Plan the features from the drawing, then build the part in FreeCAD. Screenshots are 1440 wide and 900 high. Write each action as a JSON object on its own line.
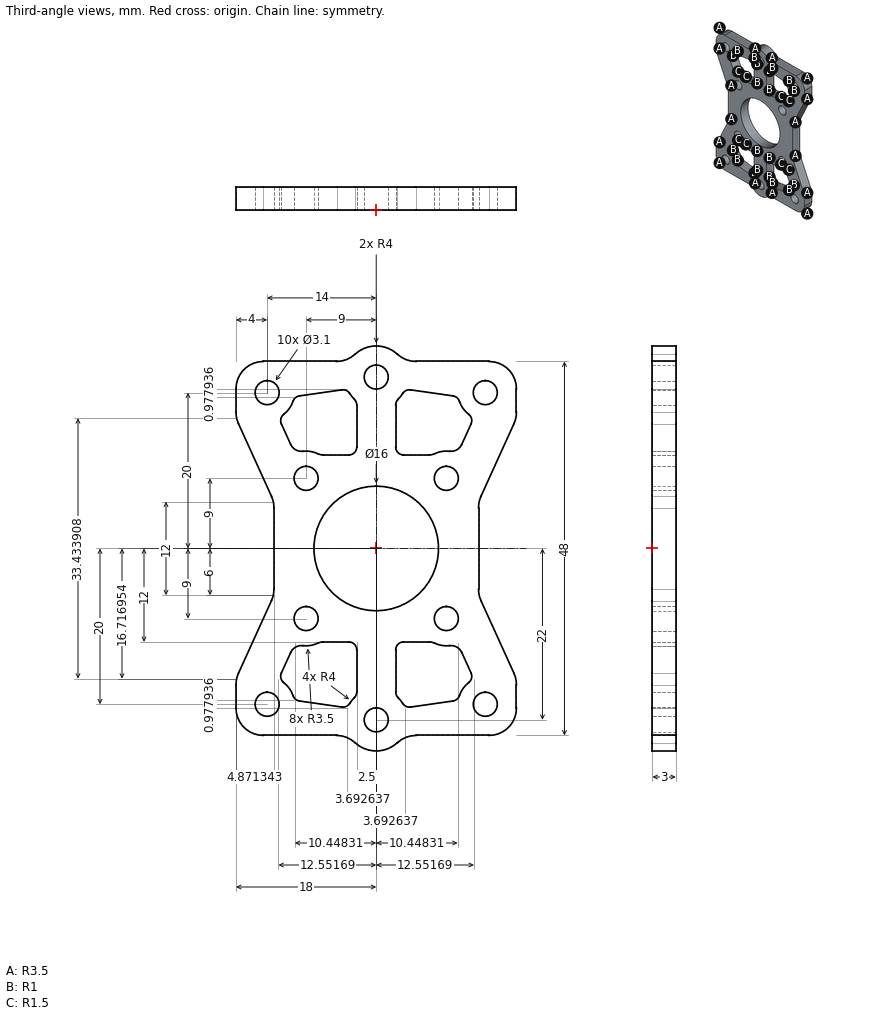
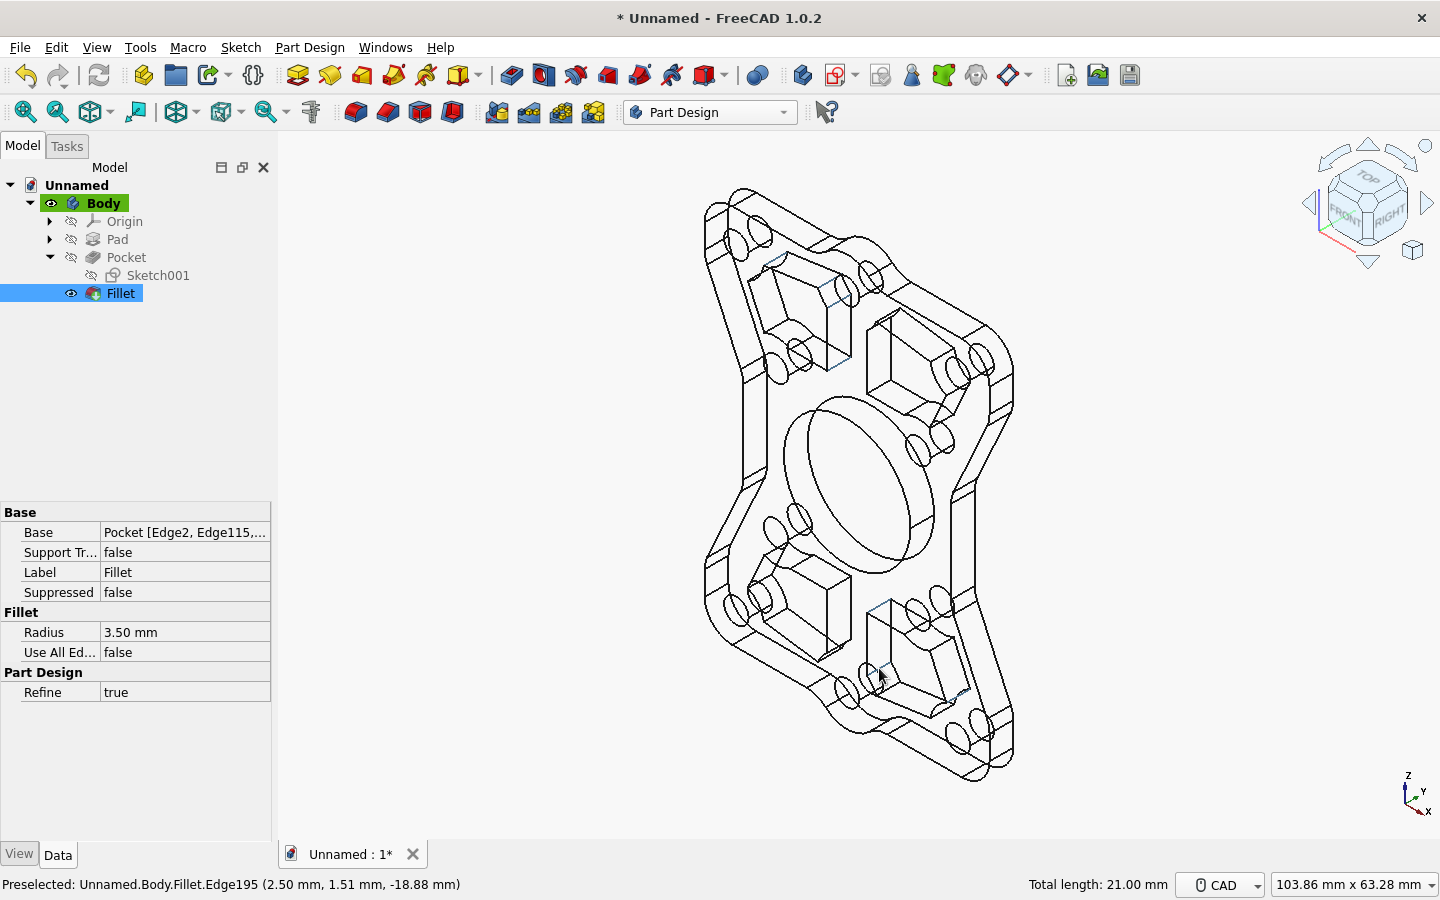
{"action": "left_click", "coordinate": [888, 688], "text": "ctrl"}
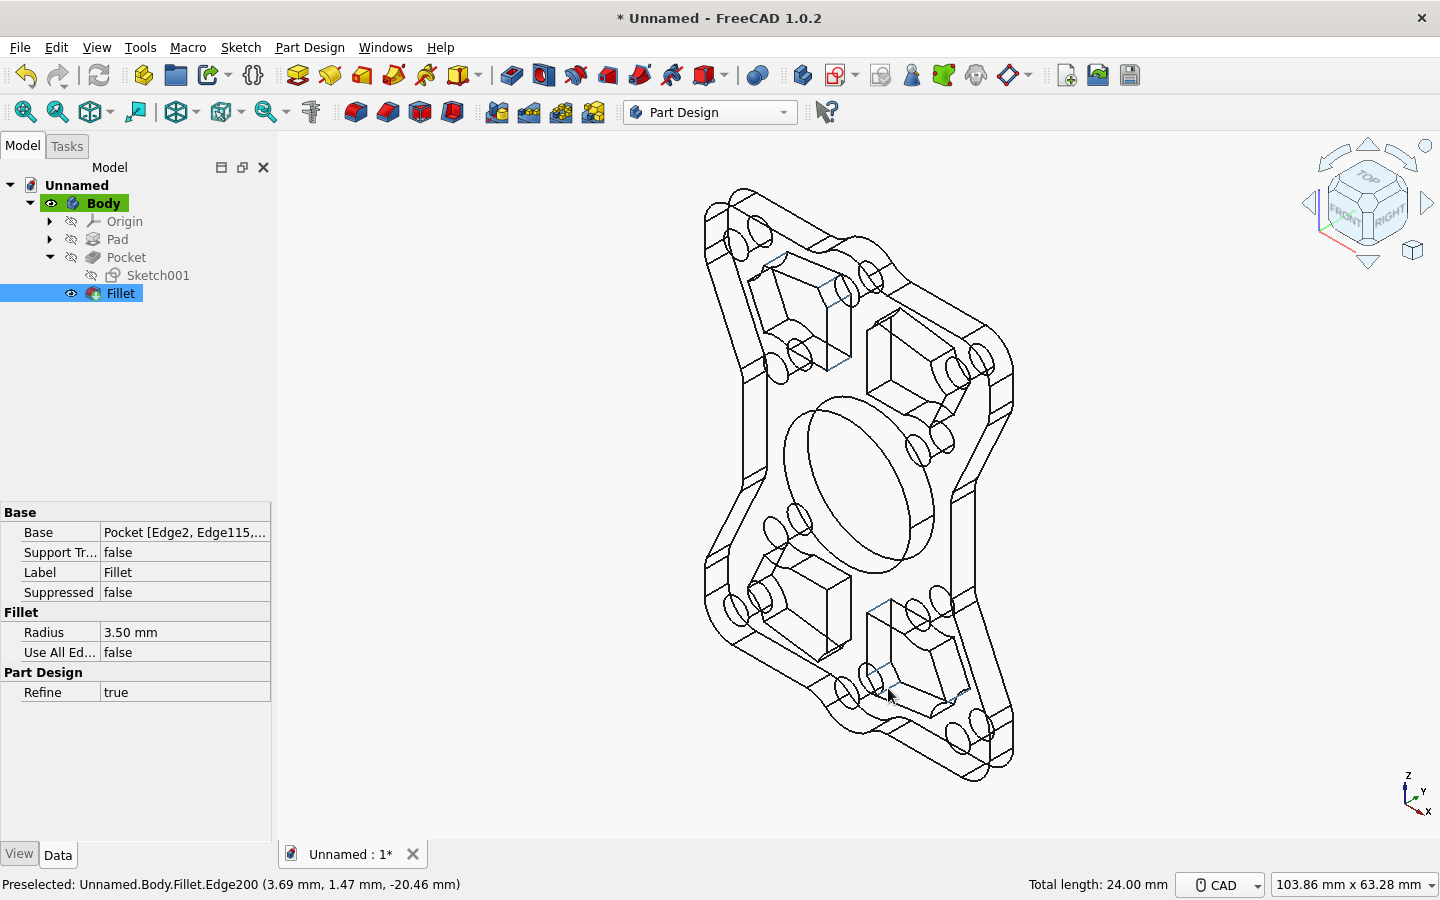
{"action": "left_click", "coordinate": [942, 710], "text": "ctrl"}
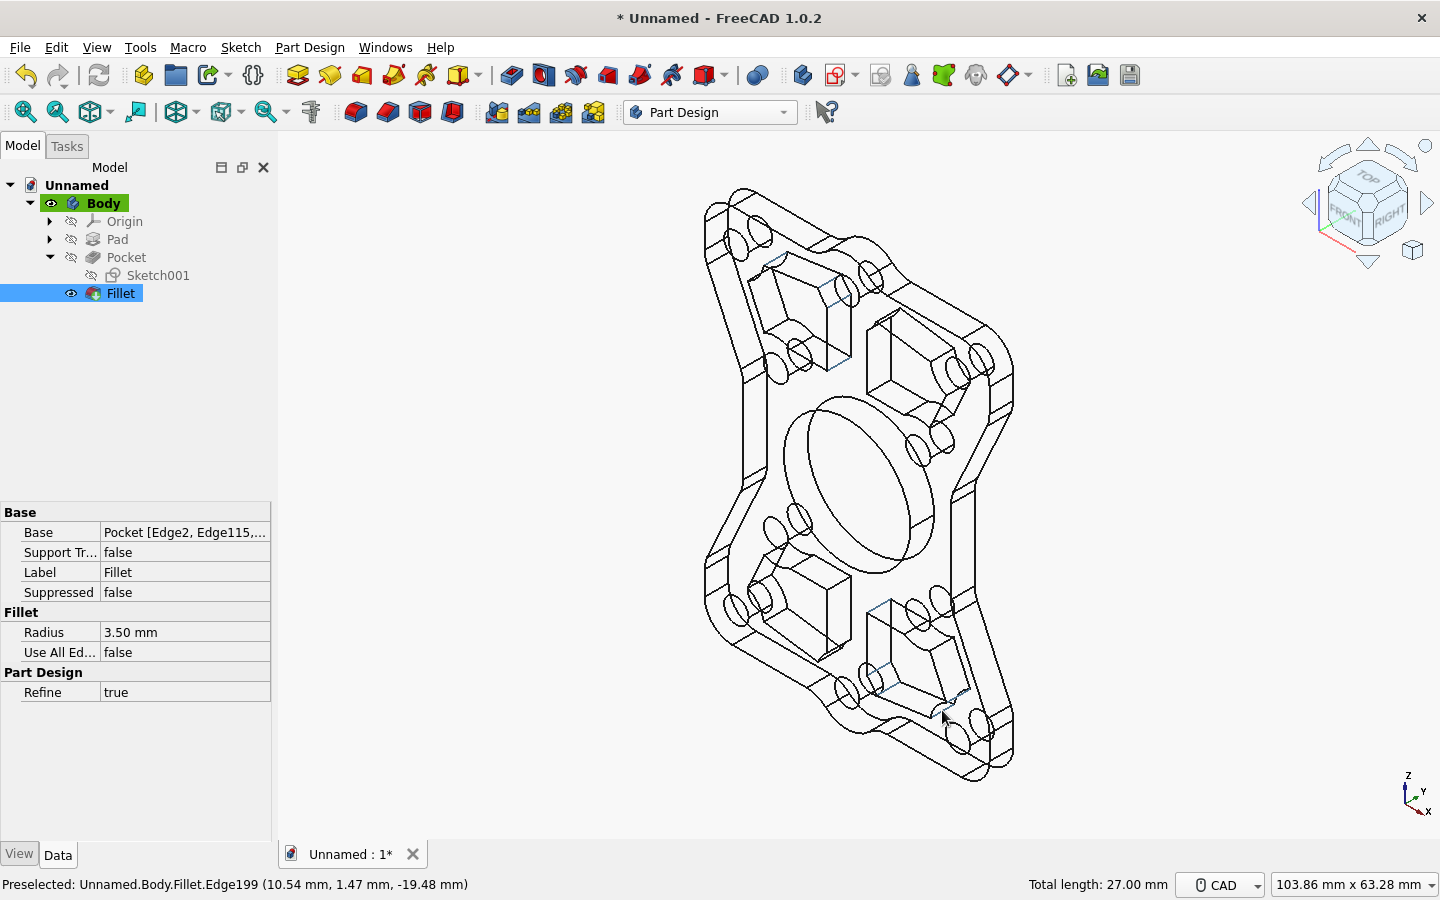
{"action": "left_click", "coordinate": [879, 386], "text": "ctrl"}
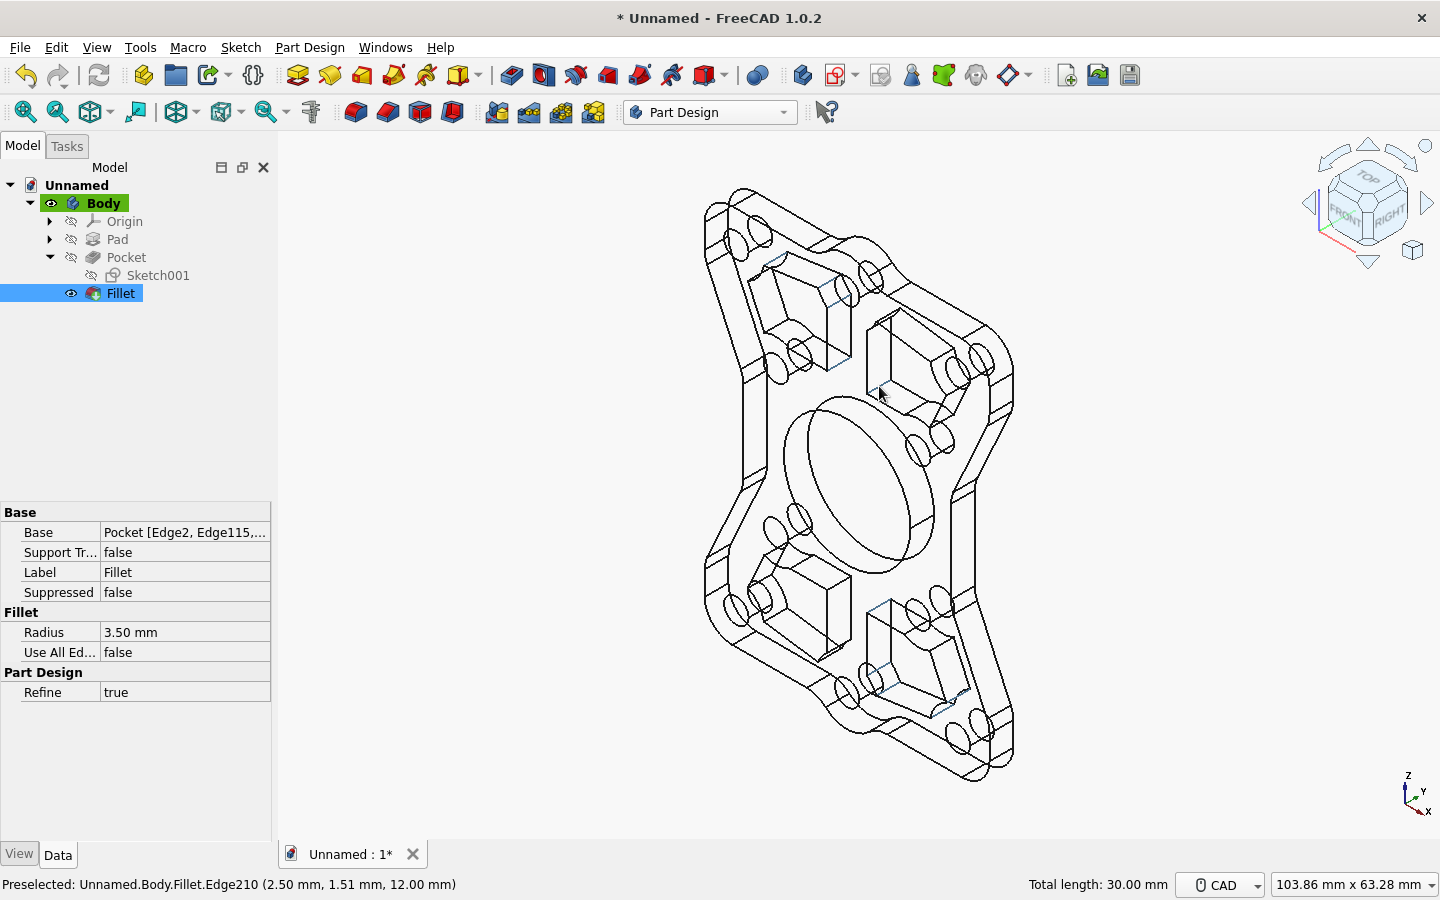
{"action": "left_click", "coordinate": [942, 354], "text": "ctrl"}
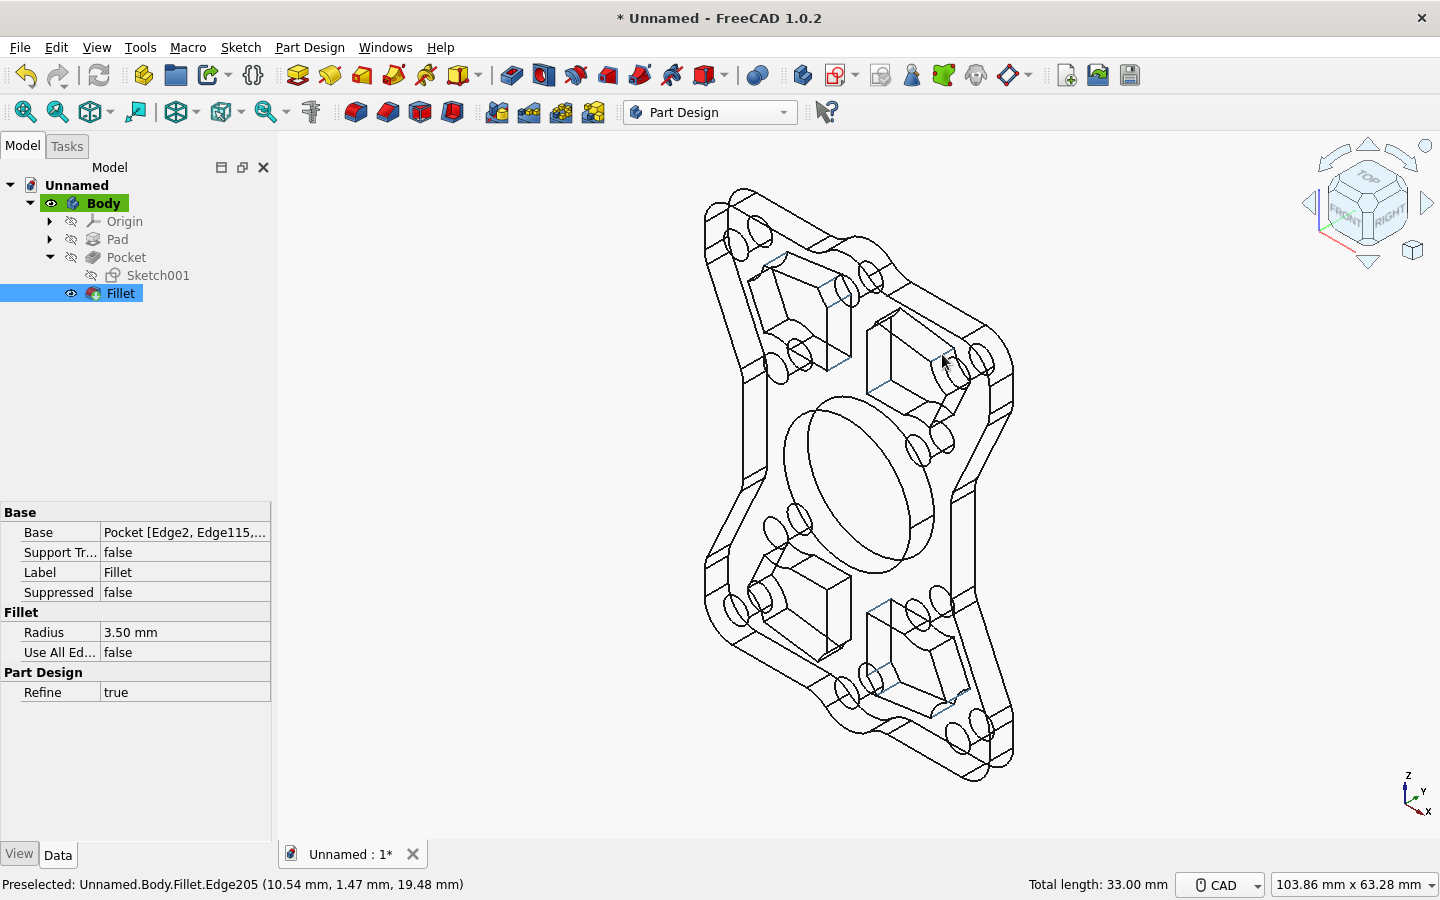
{"action": "left_click", "coordinate": [888, 314], "text": "ctrl"}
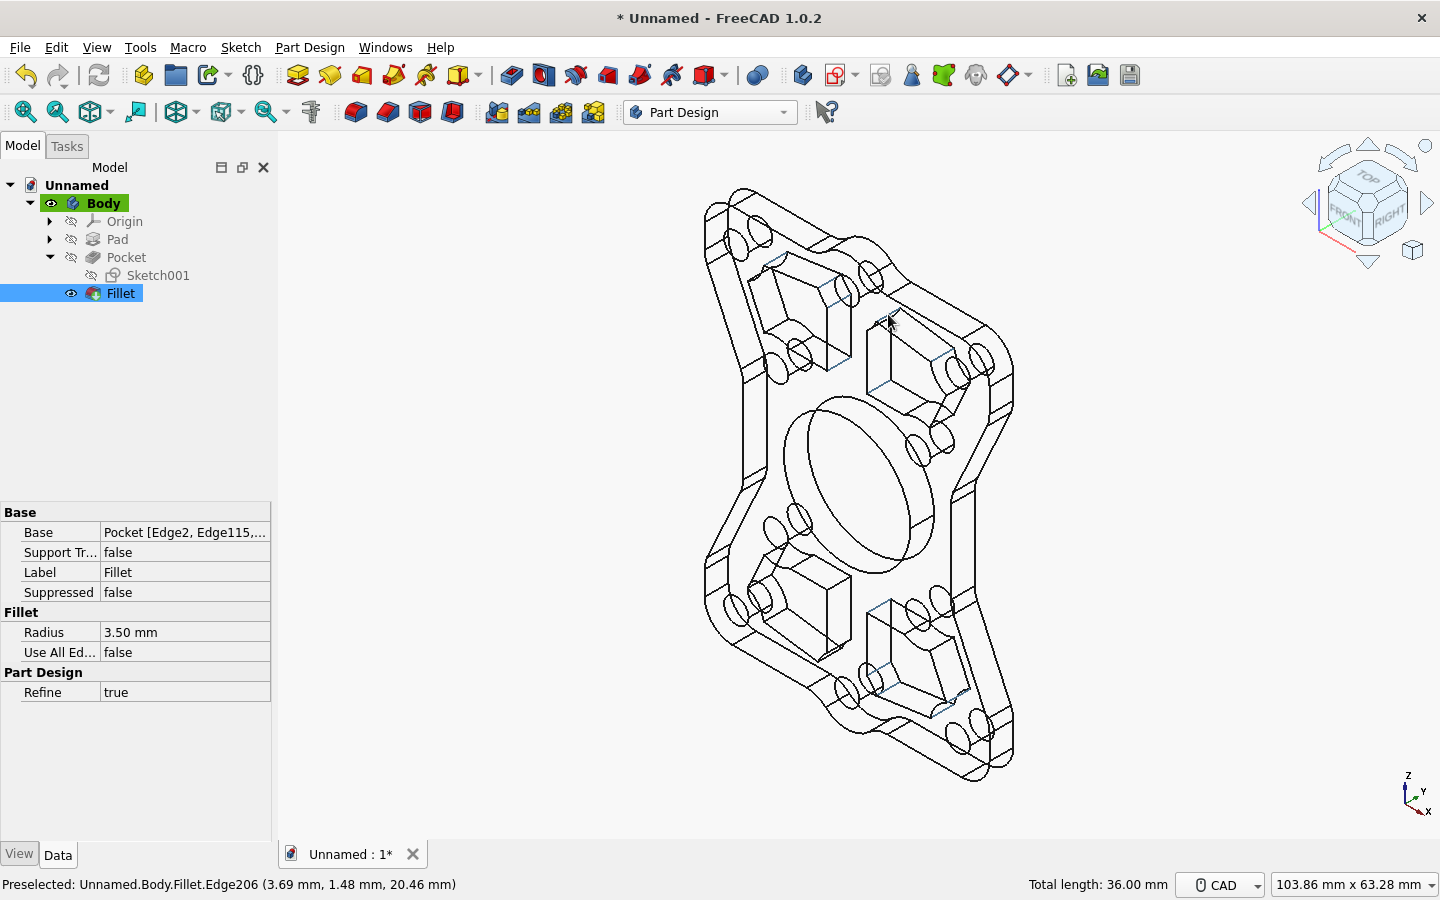
{"action": "left_click", "coordinate": [839, 645], "text": "ctrl"}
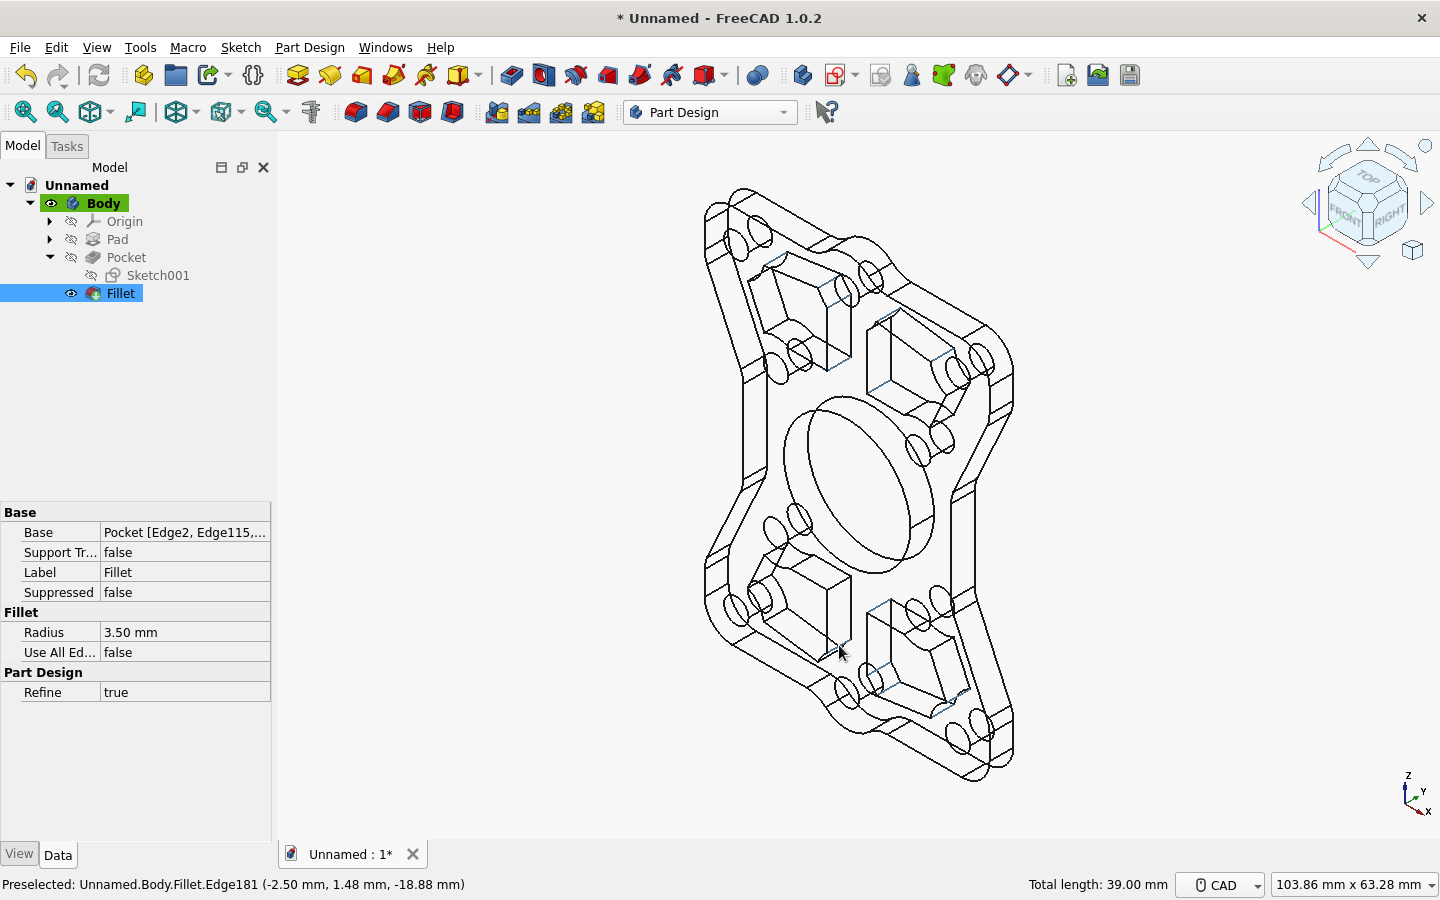
{"action": "left_click", "coordinate": [839, 582], "text": "ctrl"}